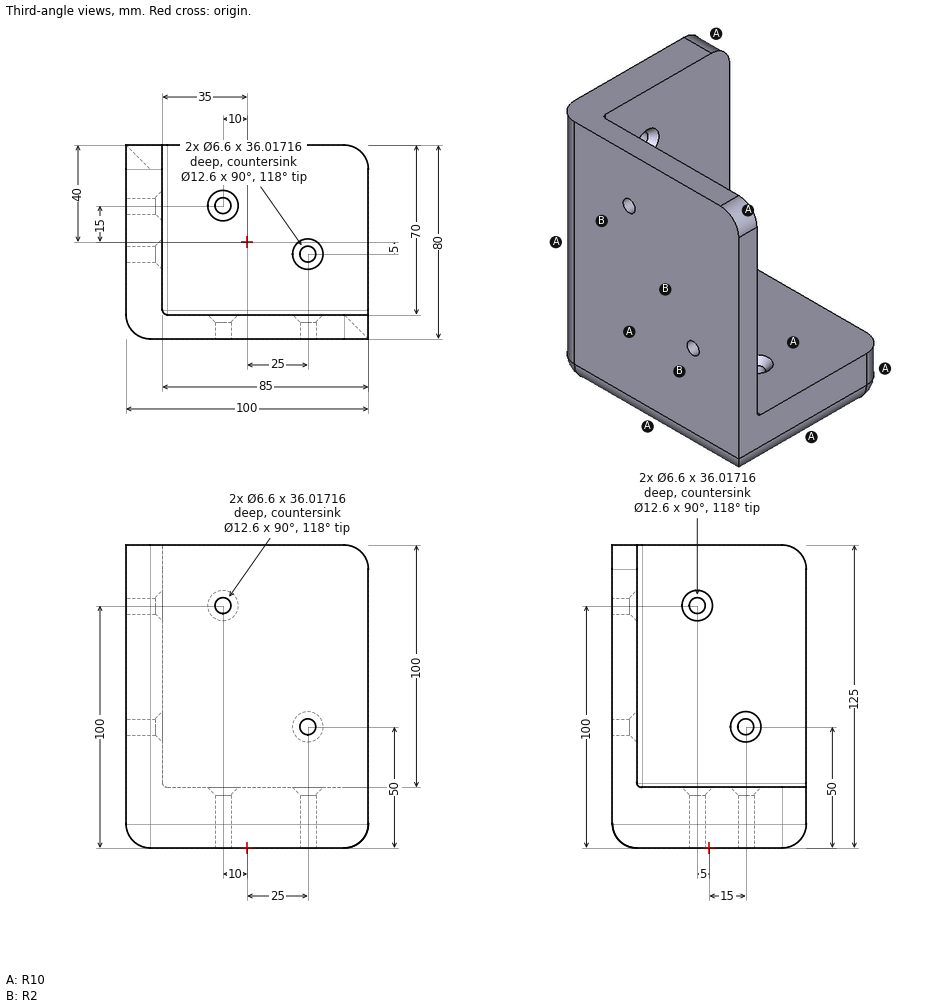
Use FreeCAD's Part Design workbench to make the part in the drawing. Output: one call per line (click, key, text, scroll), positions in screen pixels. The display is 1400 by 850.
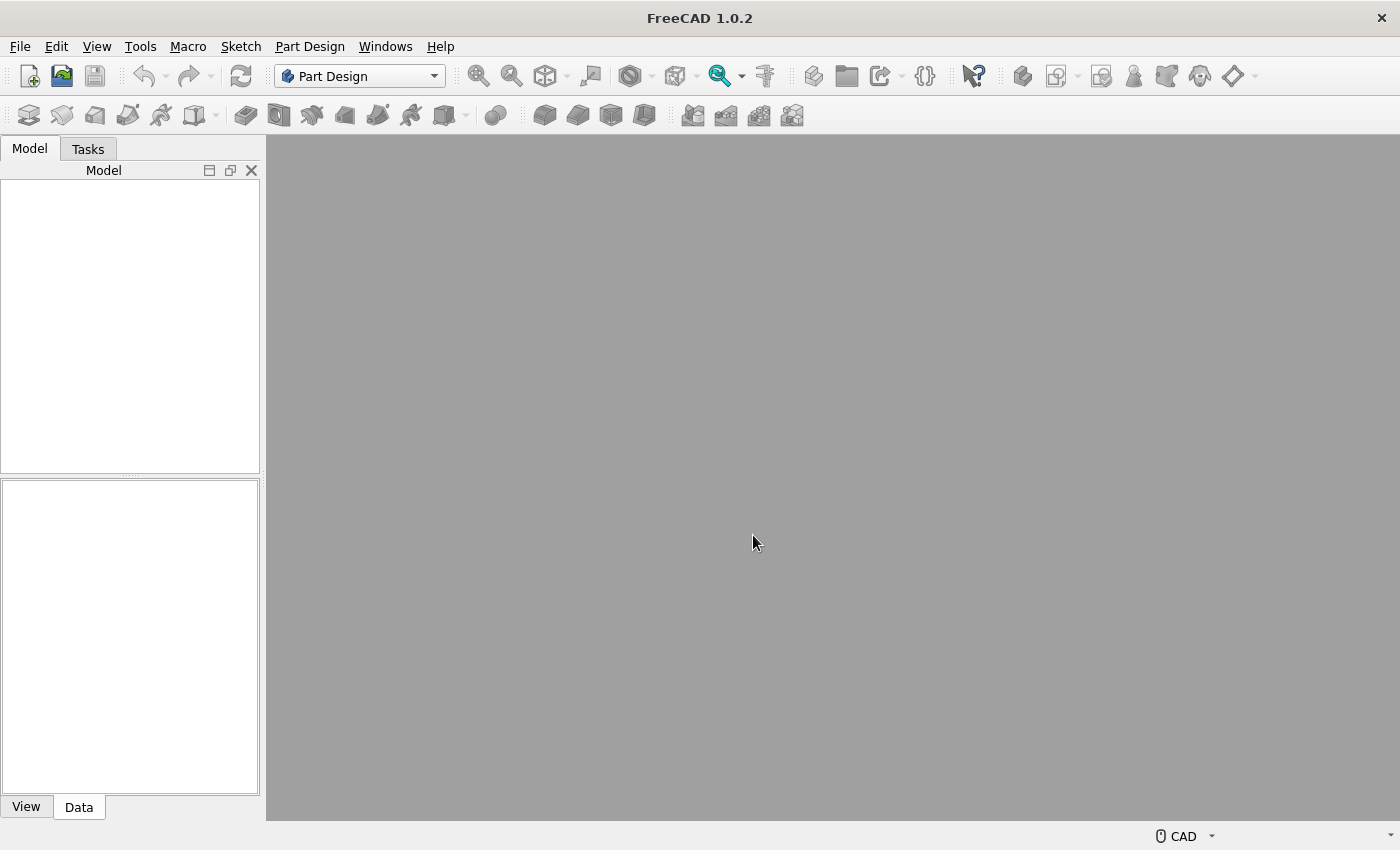
click(29, 76)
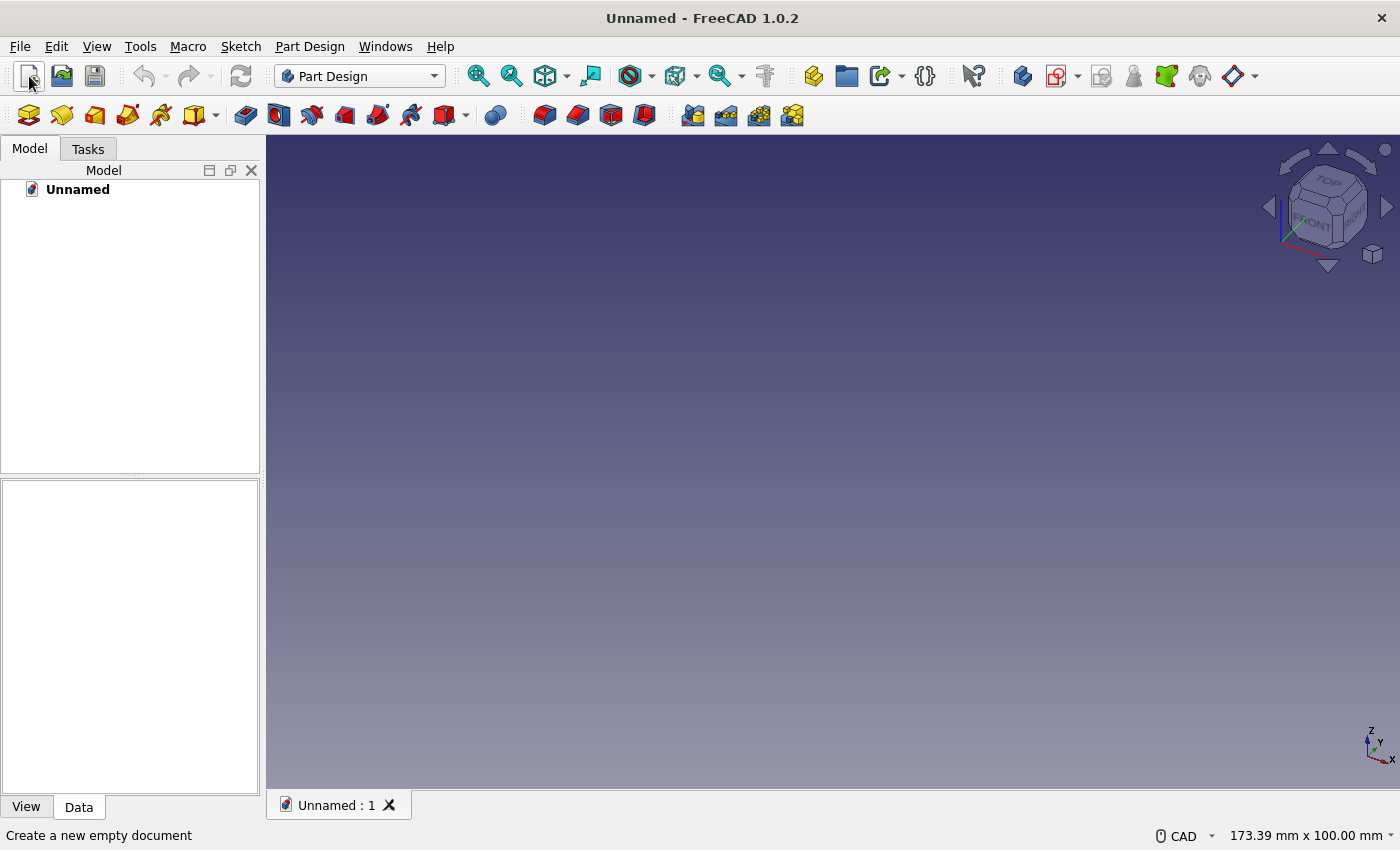
click(1056, 76)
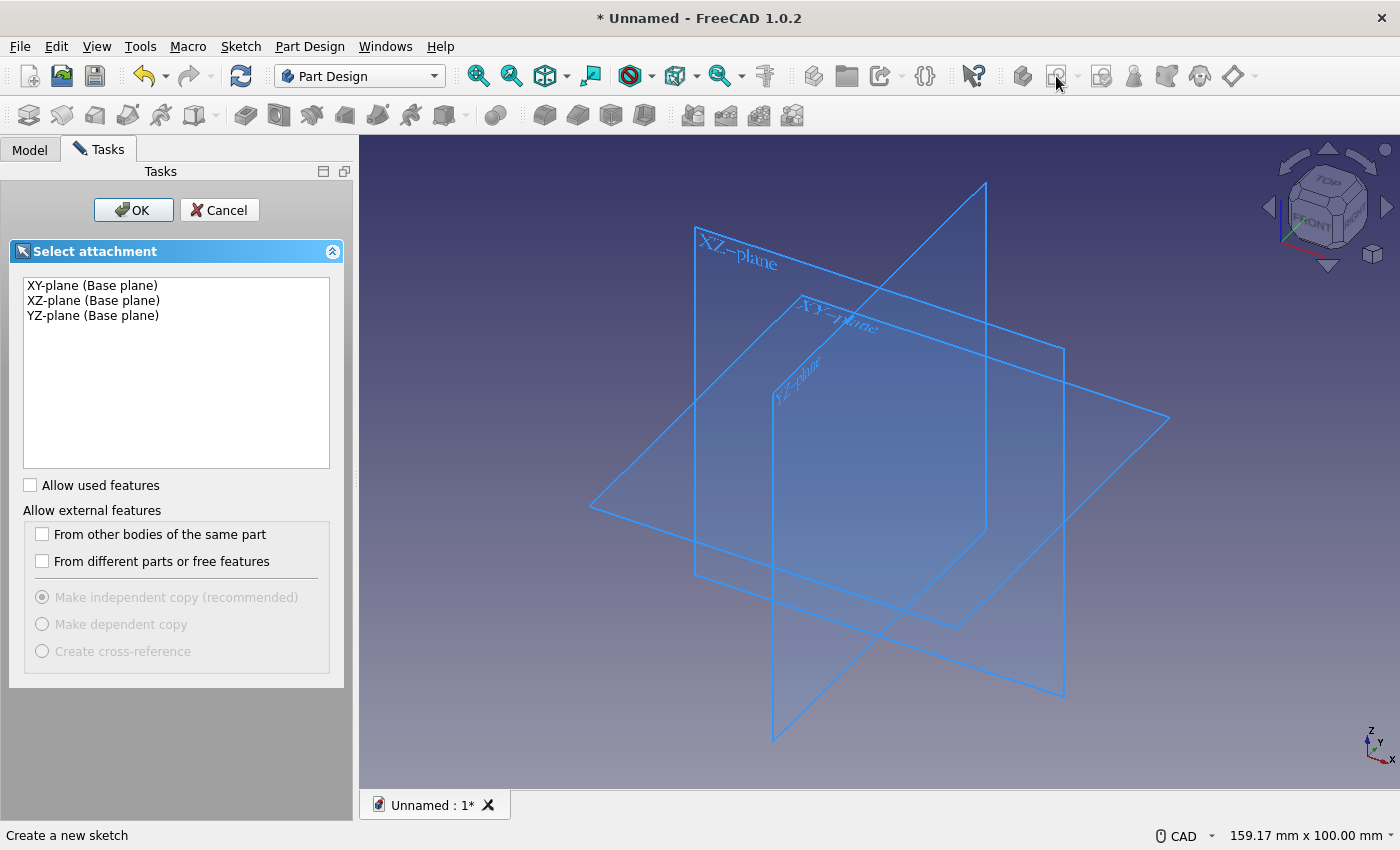
click(84, 286)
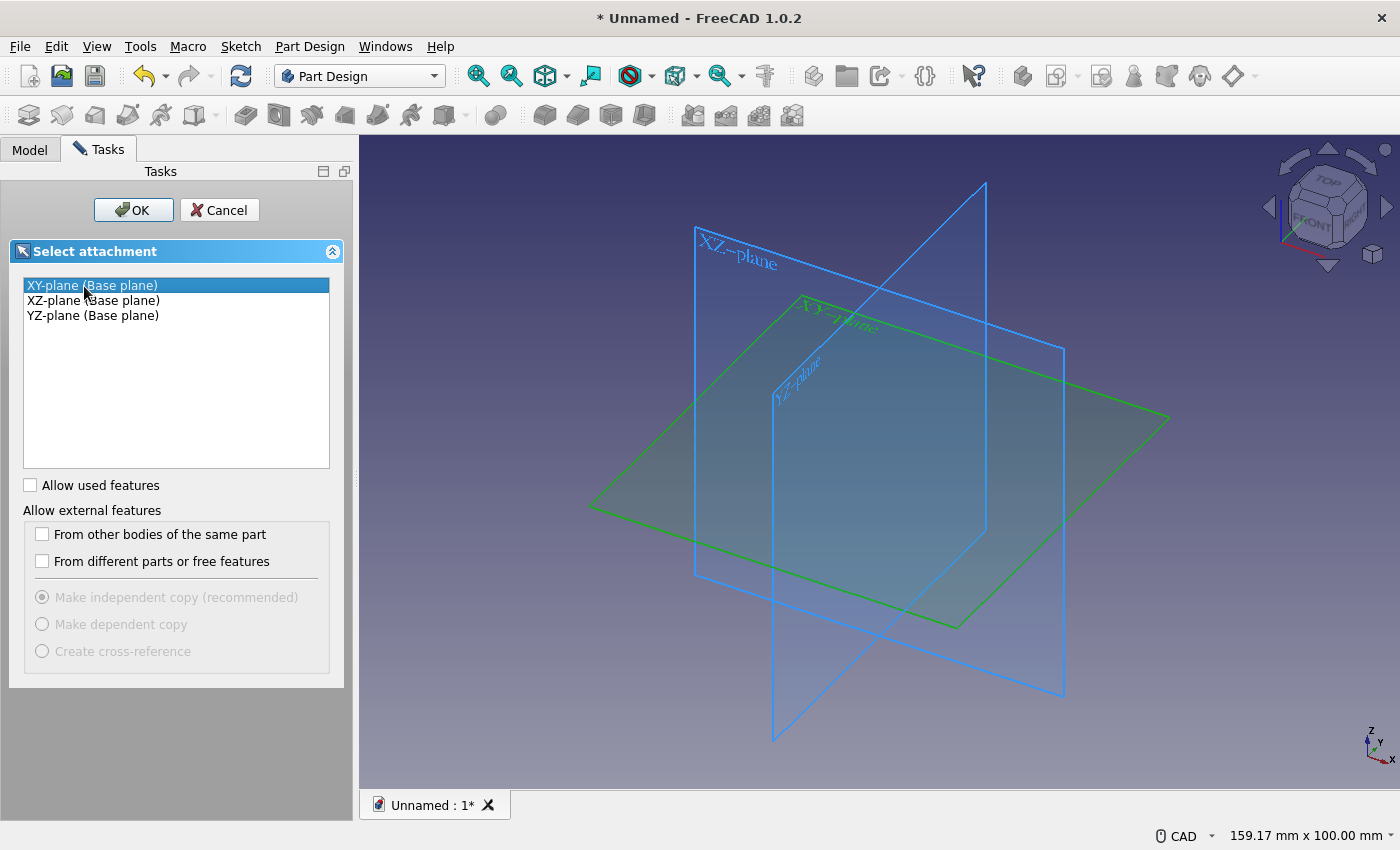
click(134, 210)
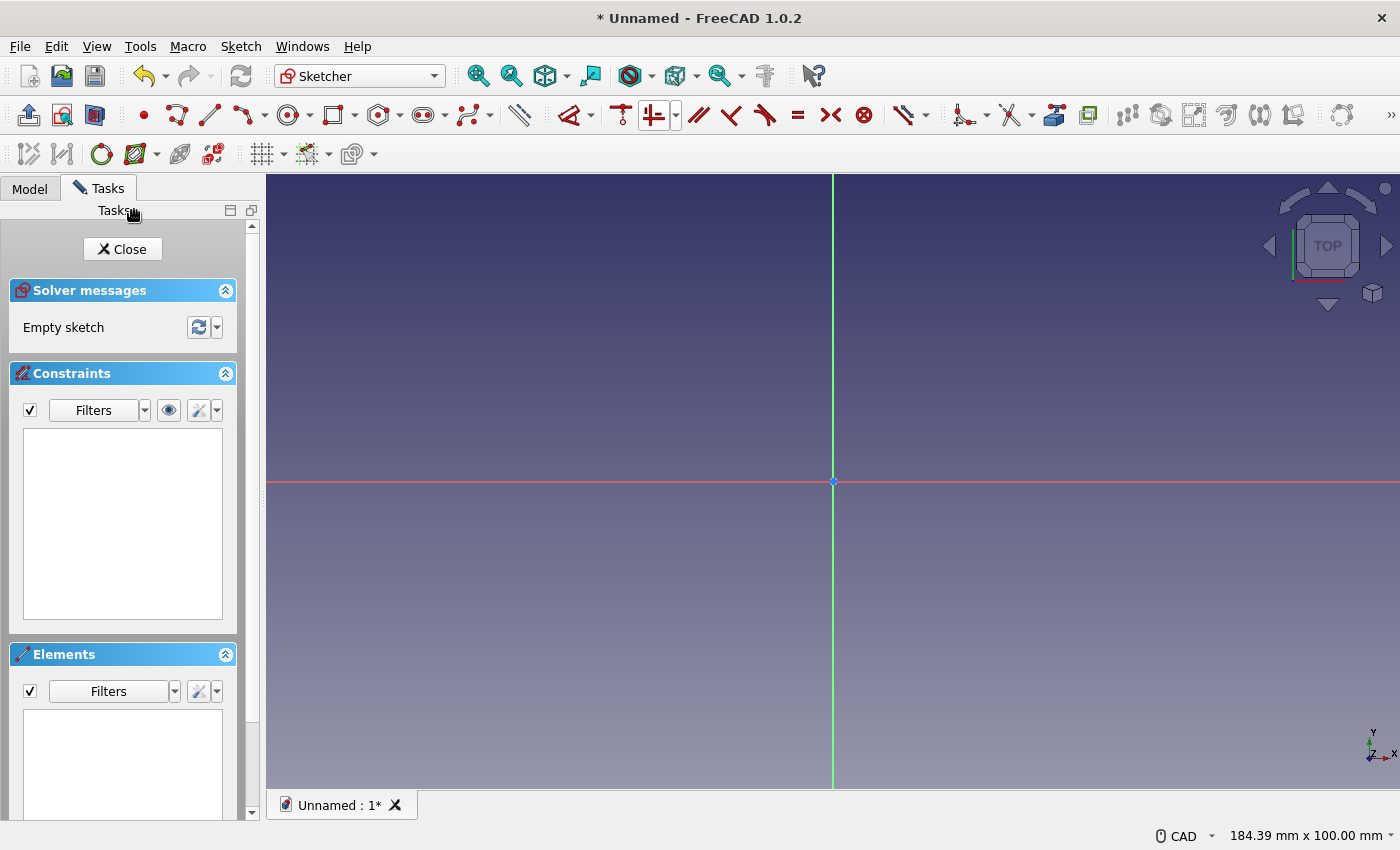
click(354, 116)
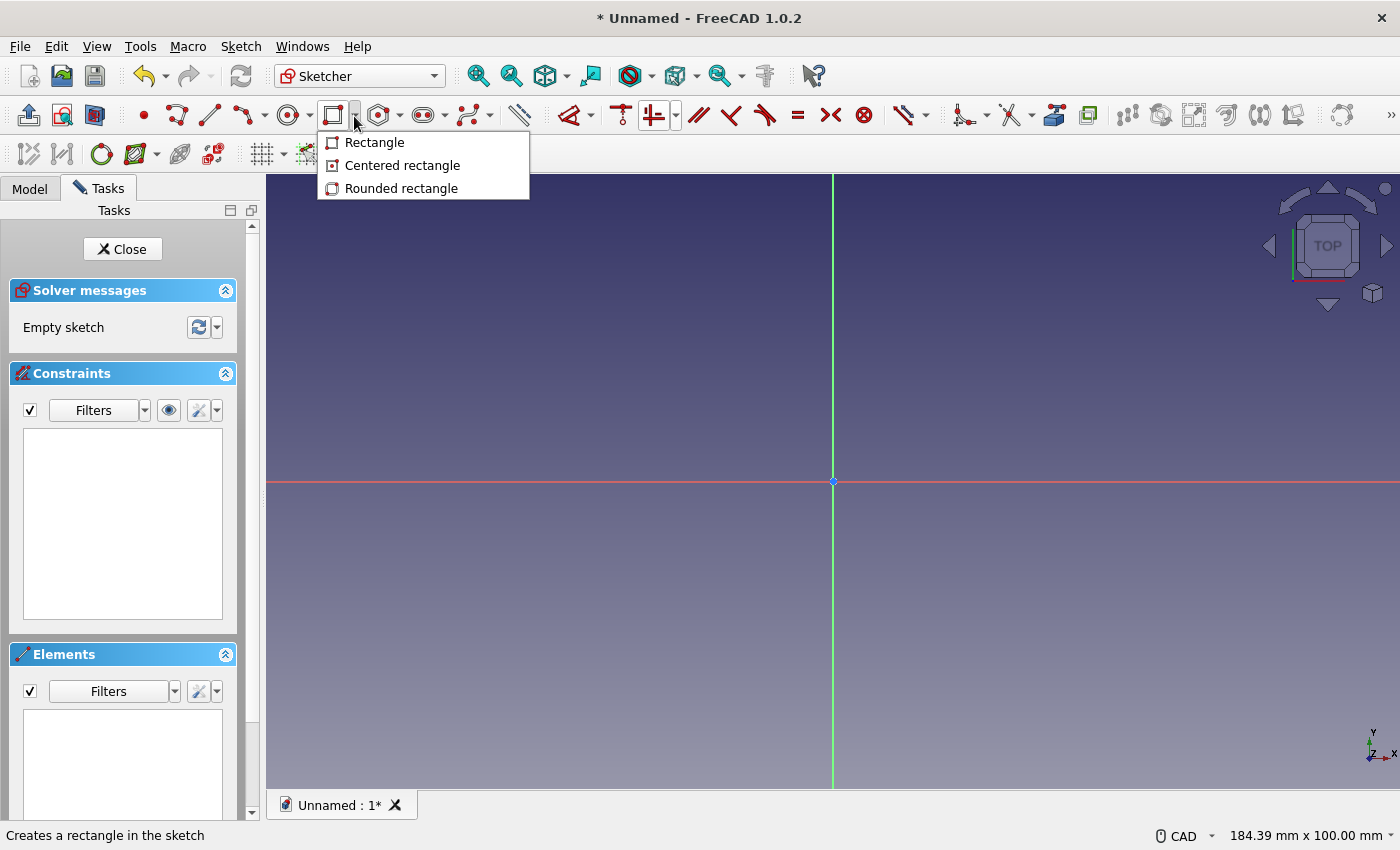
click(424, 166)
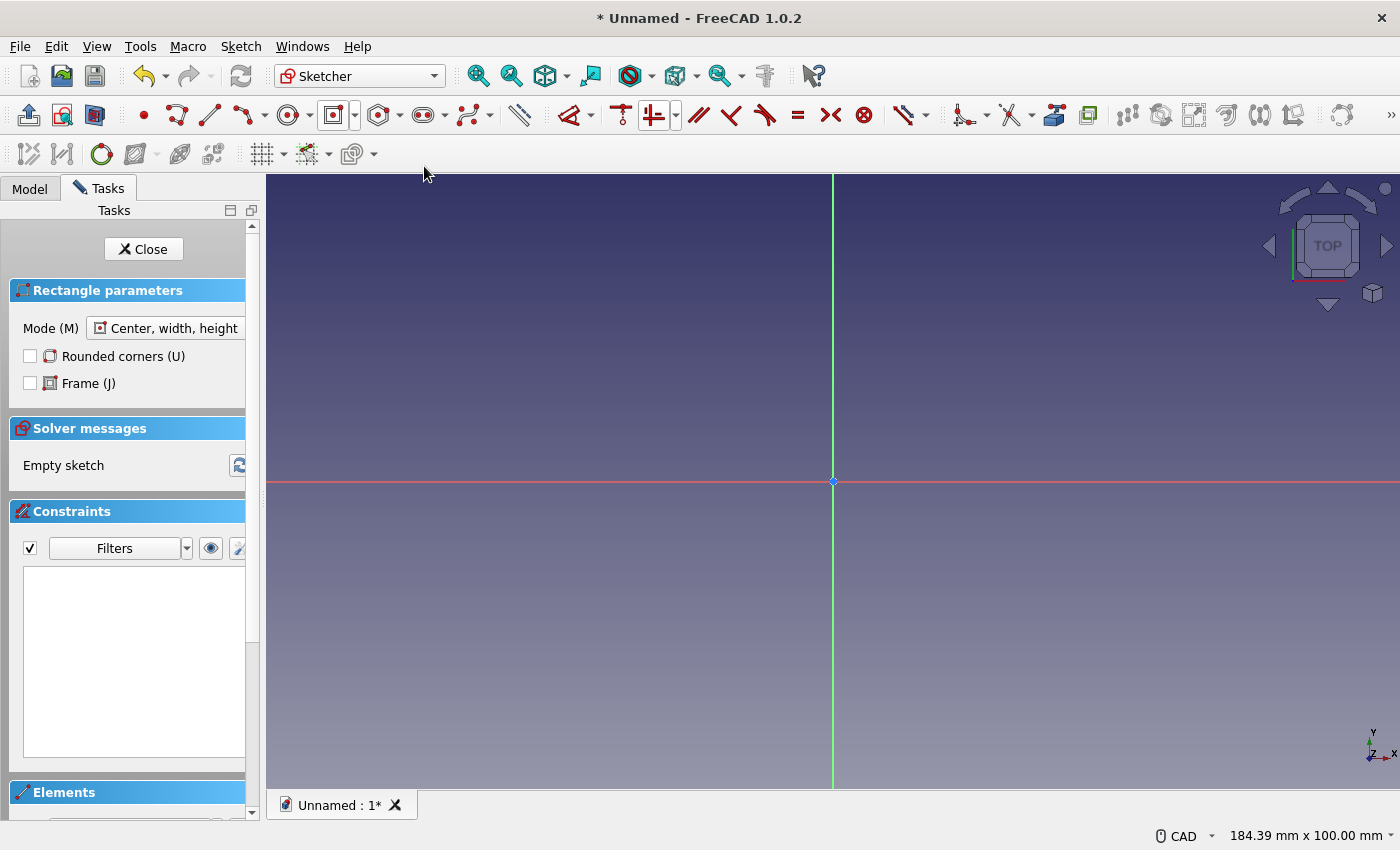
click(833, 482)
move(1140, 236)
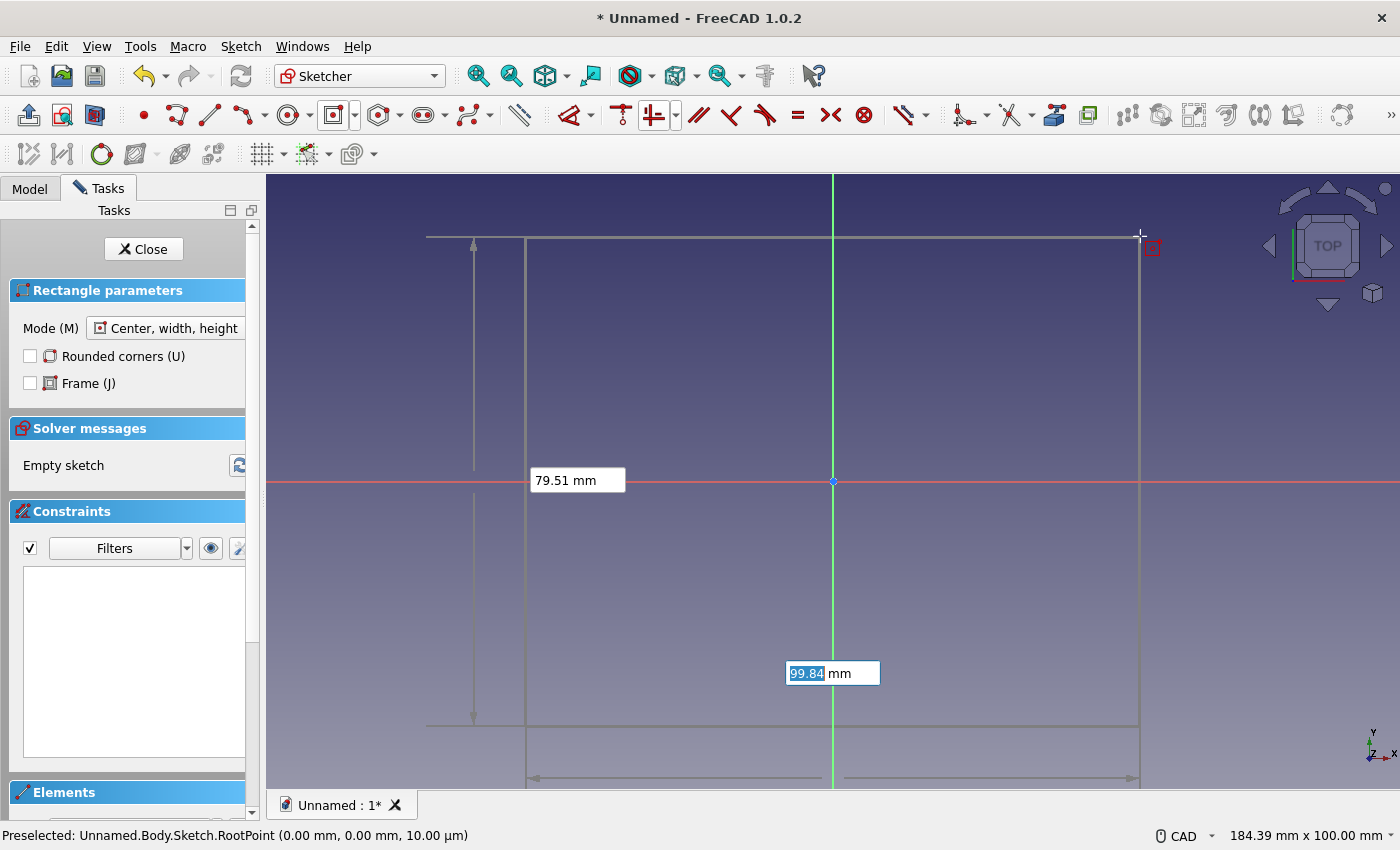
text(100)
key(Tab)
text(80)
key(Return)
key(Escape)